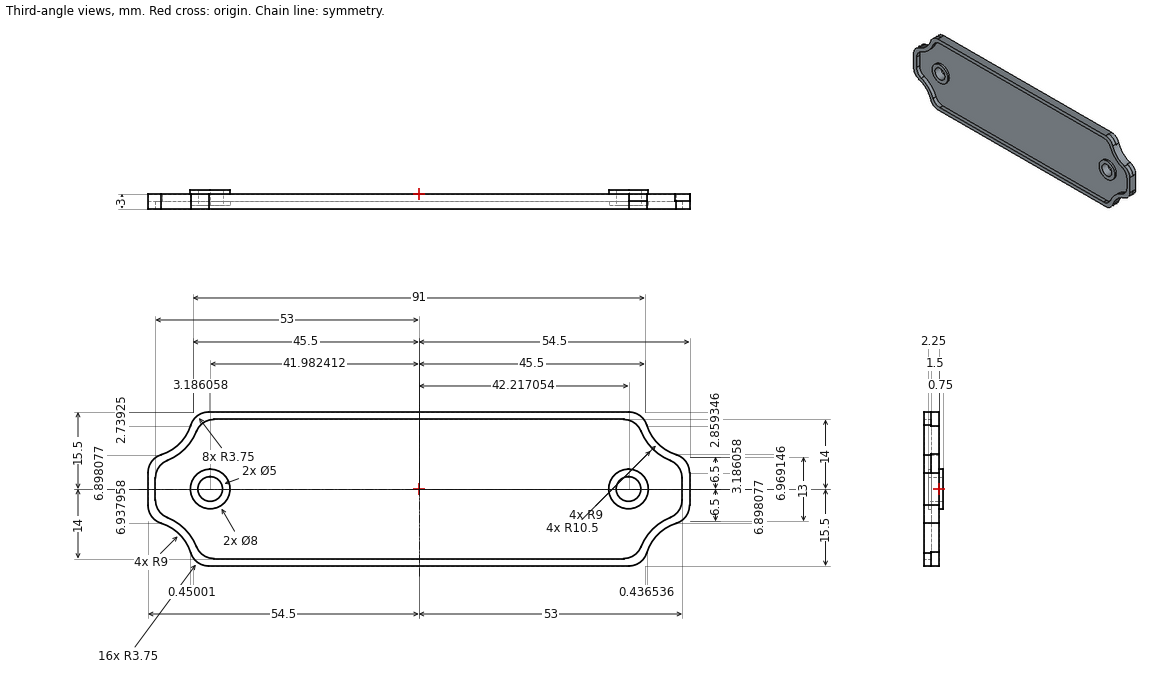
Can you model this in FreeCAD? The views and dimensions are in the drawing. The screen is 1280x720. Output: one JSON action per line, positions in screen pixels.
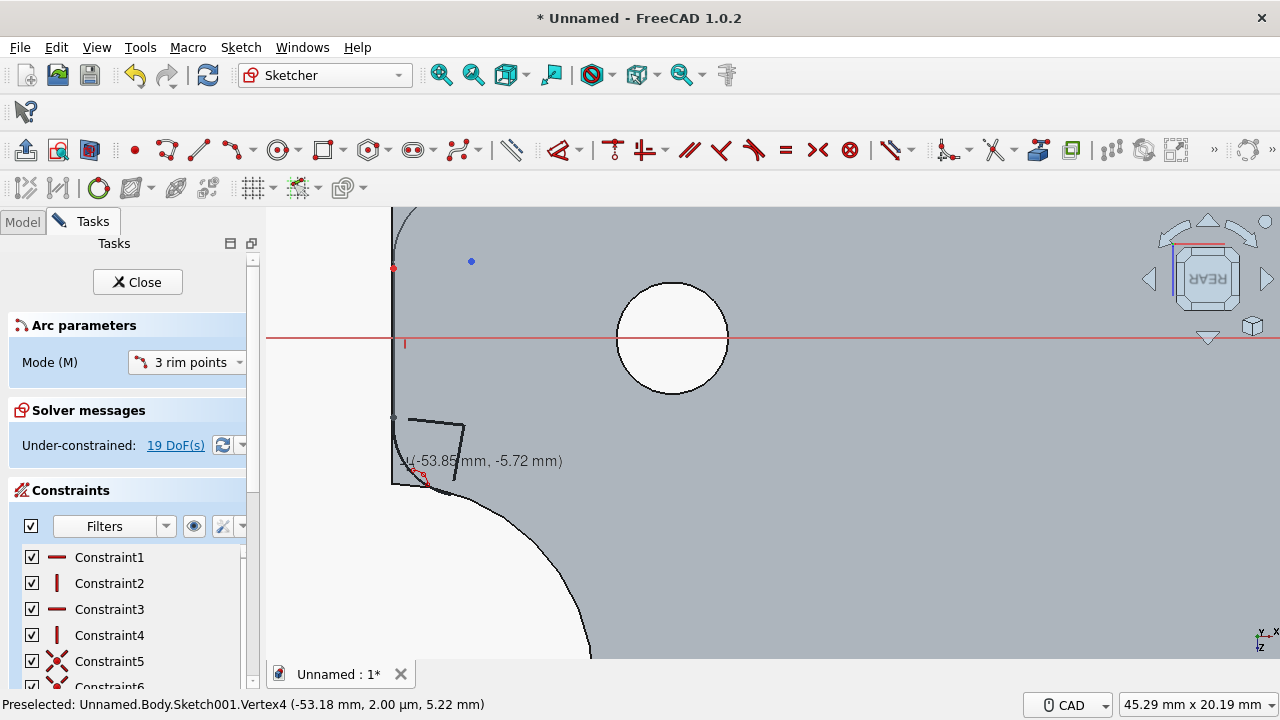
{"action": "left_click", "coordinate": [409, 462]}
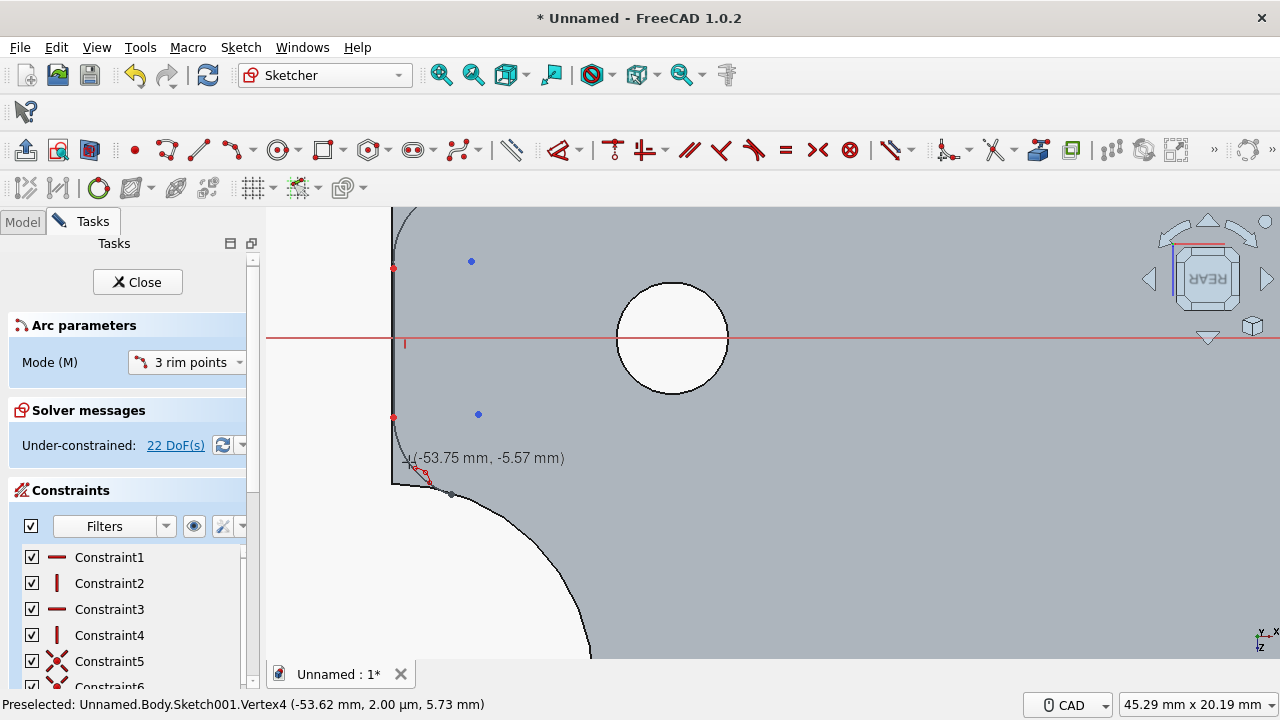
{"action": "scroll", "coordinate": [407, 464], "scroll_direction": "down", "scroll_amount": 7}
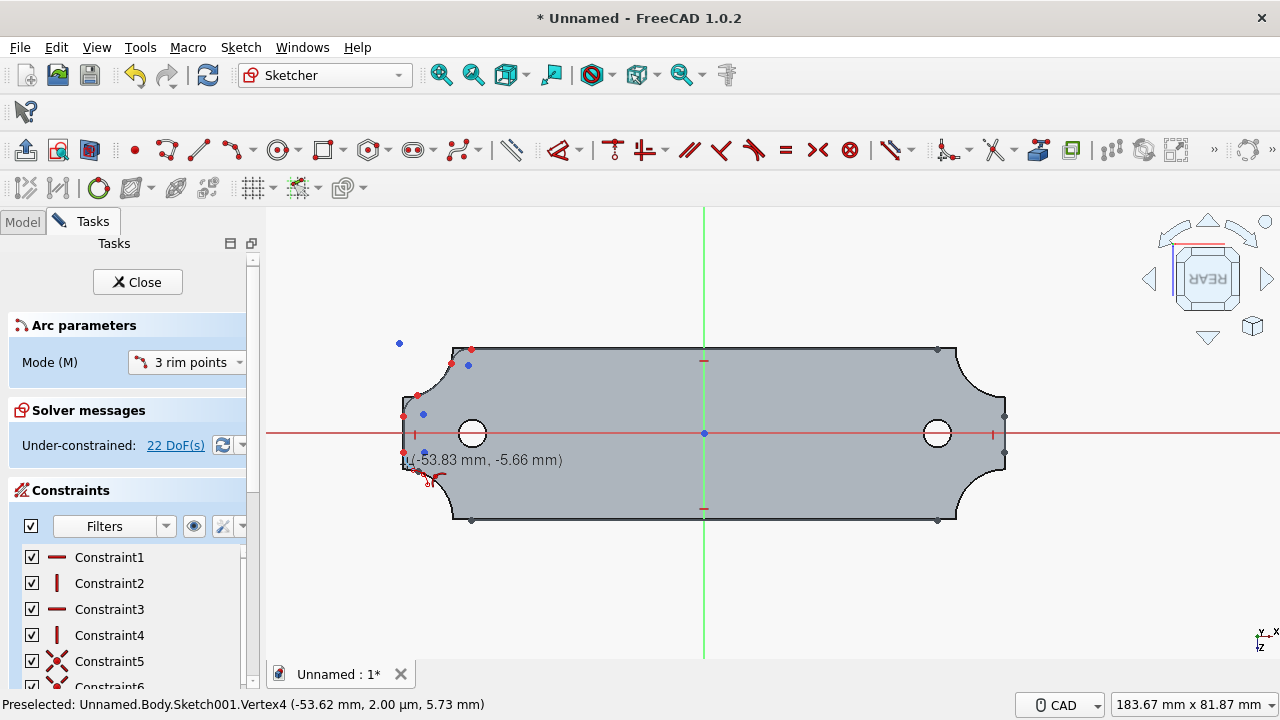
{"action": "left_click", "coordinate": [418, 472]}
{"action": "left_click", "coordinate": [451, 504]}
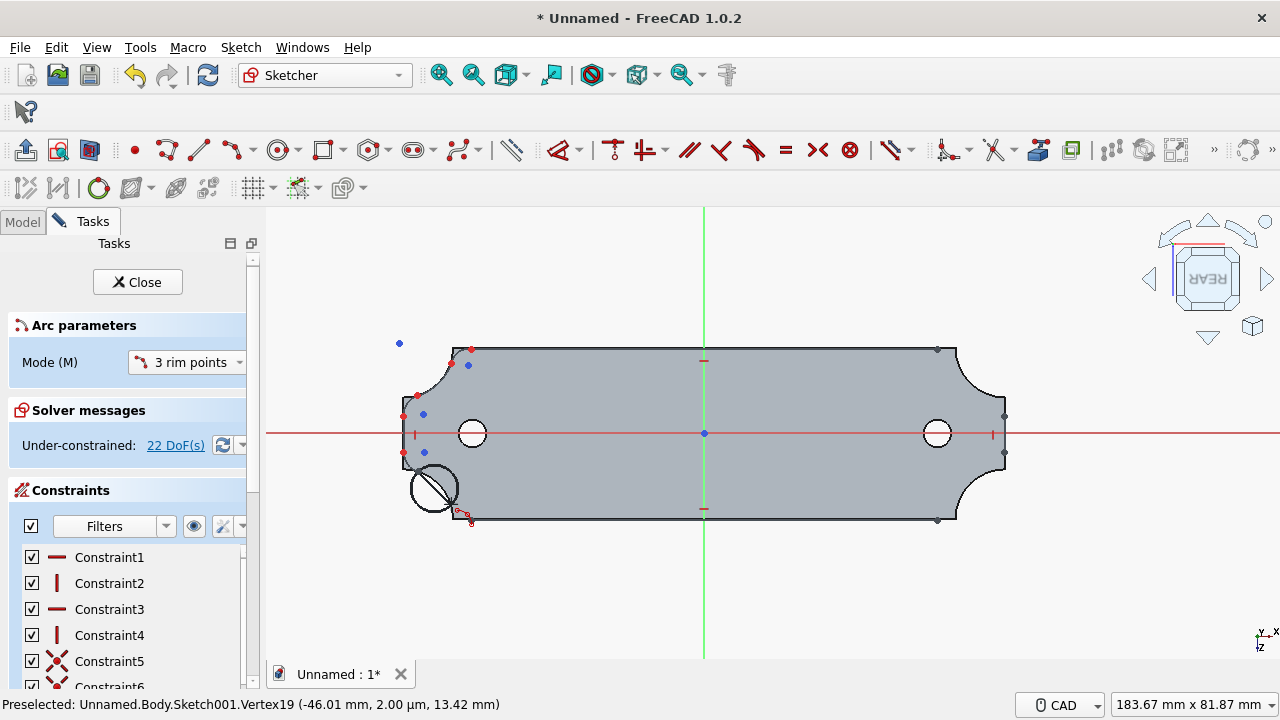
{"action": "scroll", "coordinate": [439, 484], "scroll_direction": "up", "scroll_amount": 6}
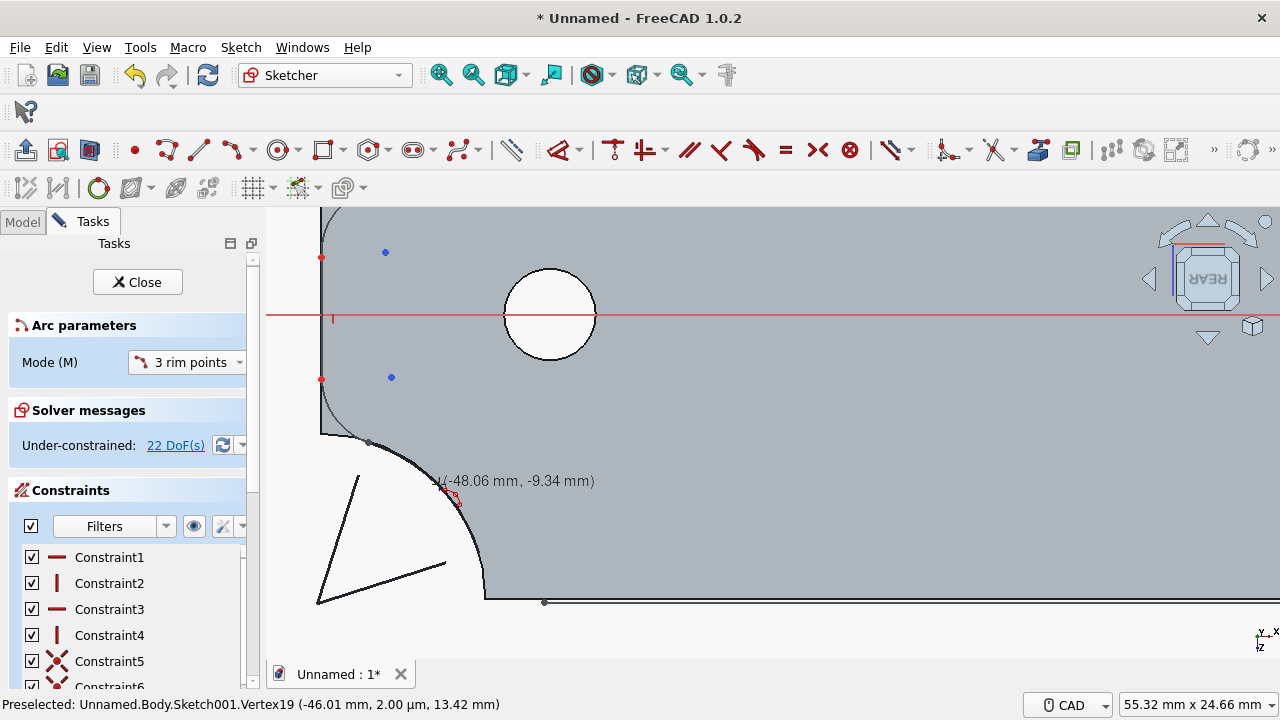
{"action": "left_click", "coordinate": [437, 482]}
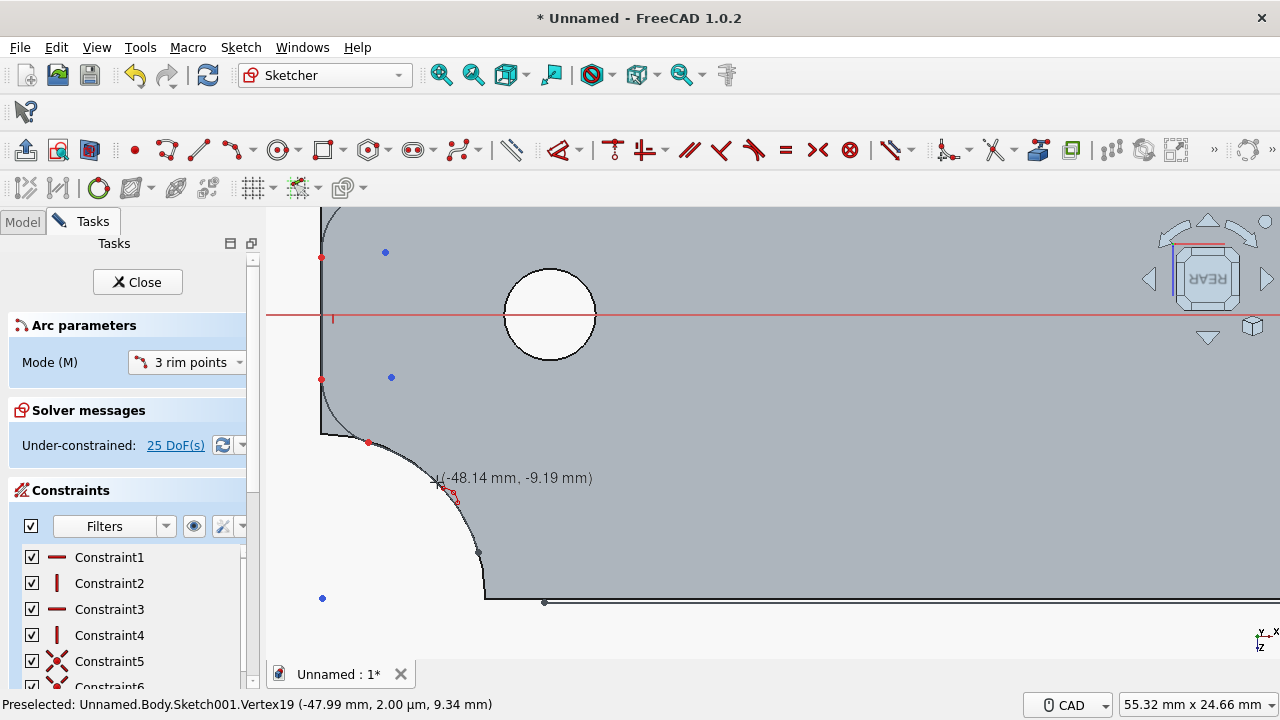
{"action": "scroll", "coordinate": [439, 484], "scroll_direction": "down", "scroll_amount": 6}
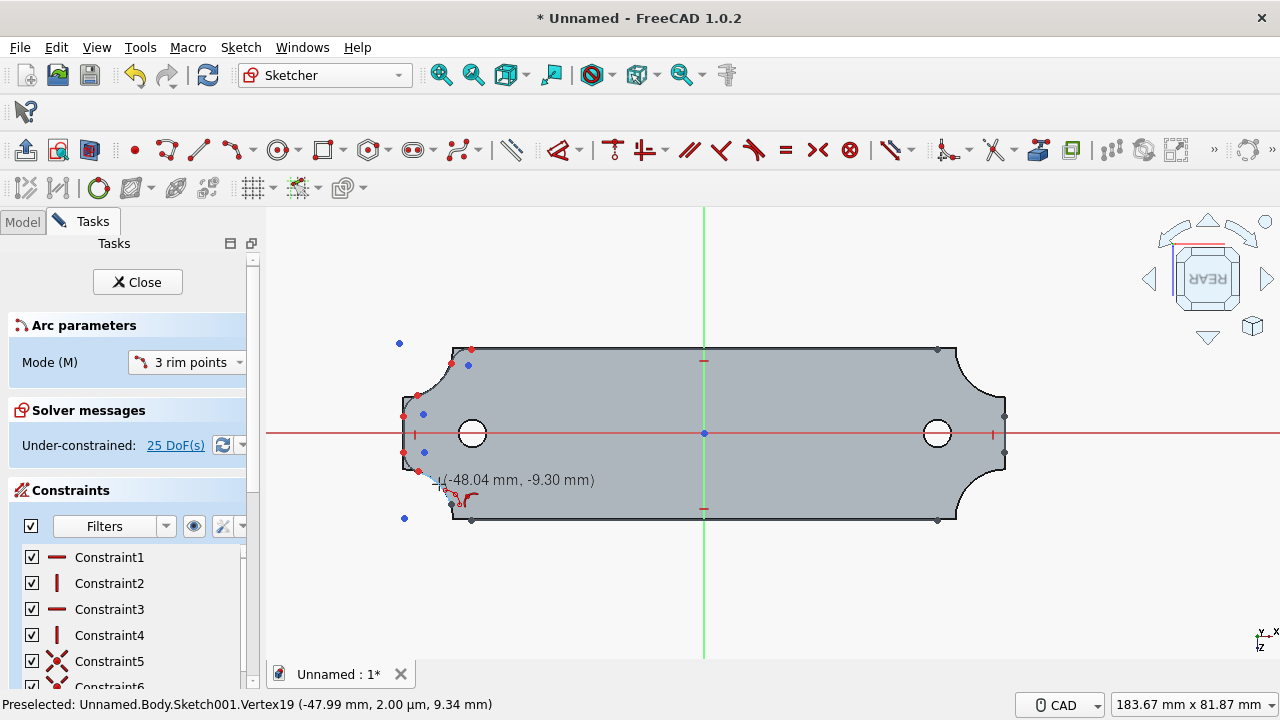
{"action": "left_click", "coordinate": [451, 505]}
{"action": "left_click", "coordinate": [471, 520]}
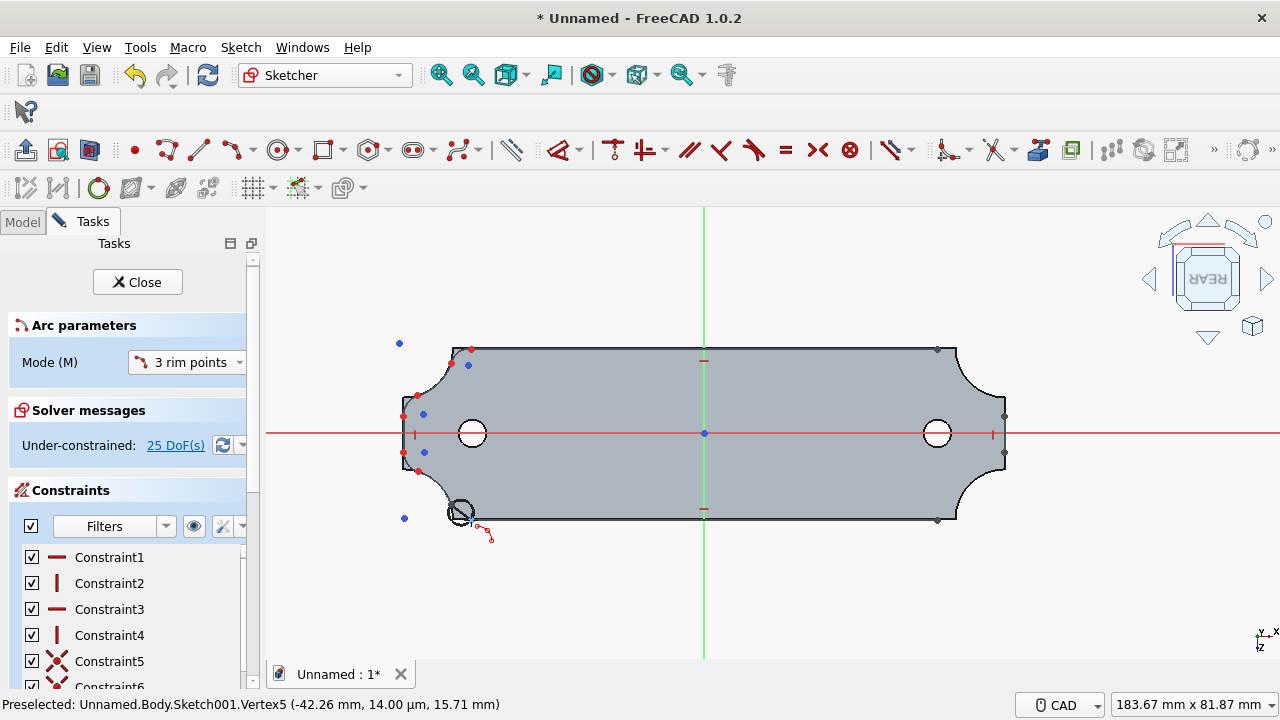
{"action": "scroll", "coordinate": [458, 515], "scroll_direction": "up", "scroll_amount": 7}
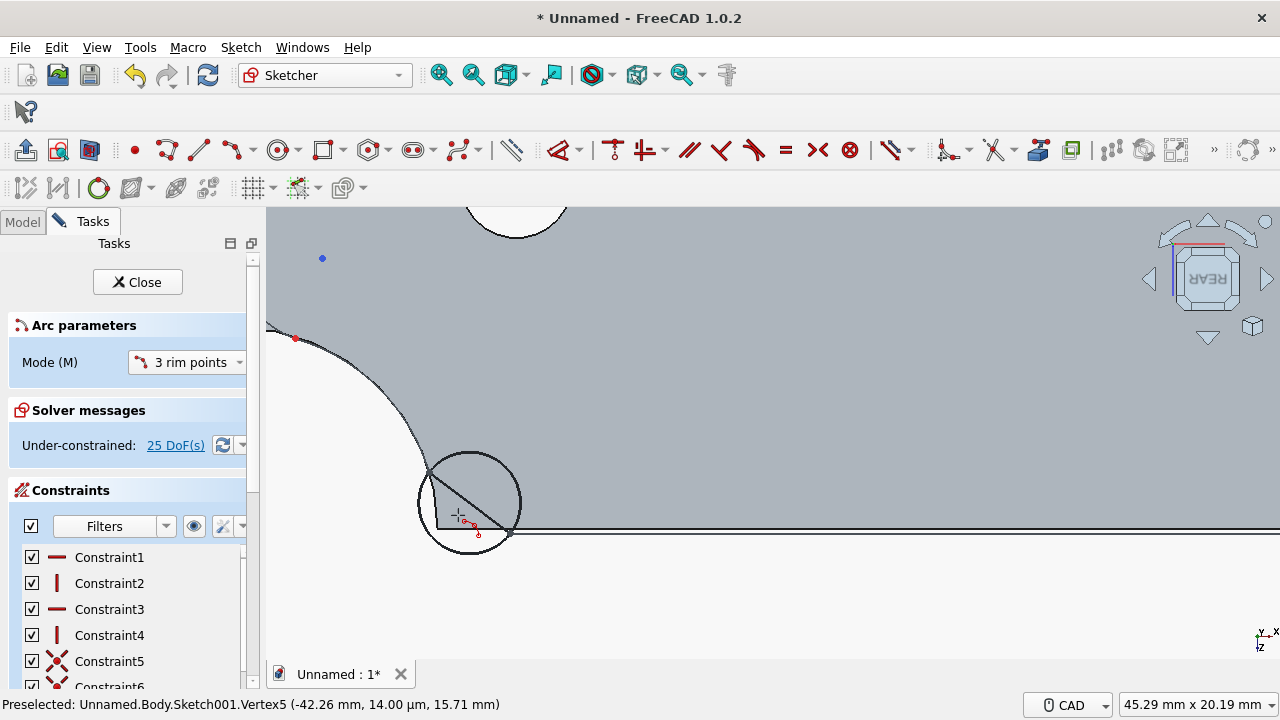
{"action": "left_click", "coordinate": [459, 513]}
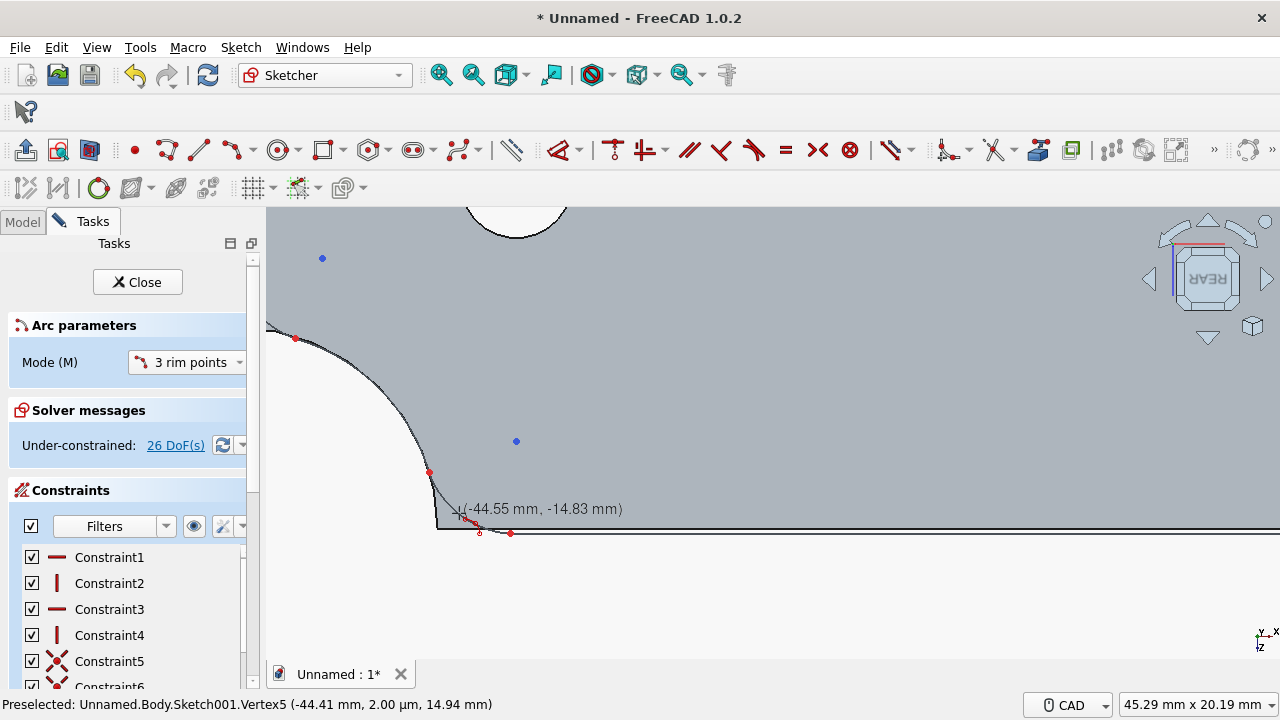
{"action": "scroll", "coordinate": [458, 515], "scroll_direction": "down", "scroll_amount": 7}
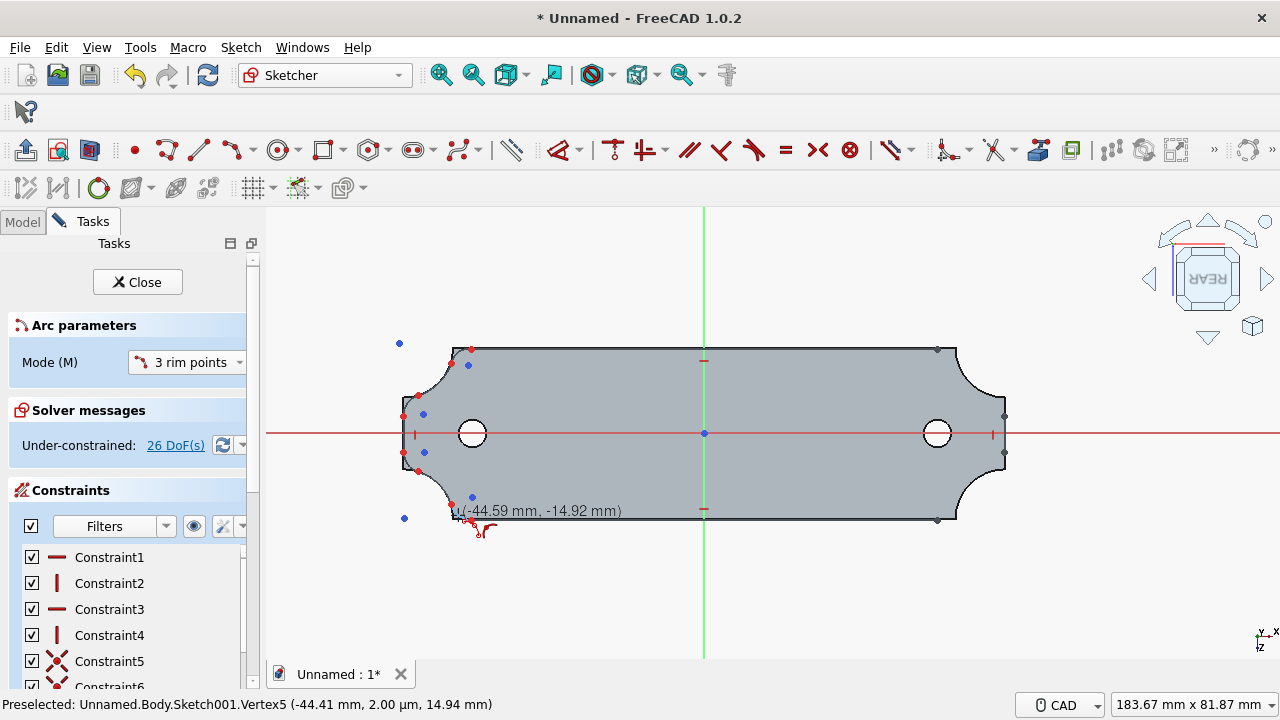
{"action": "left_click", "coordinate": [938, 520]}
{"action": "left_click", "coordinate": [958, 504]}